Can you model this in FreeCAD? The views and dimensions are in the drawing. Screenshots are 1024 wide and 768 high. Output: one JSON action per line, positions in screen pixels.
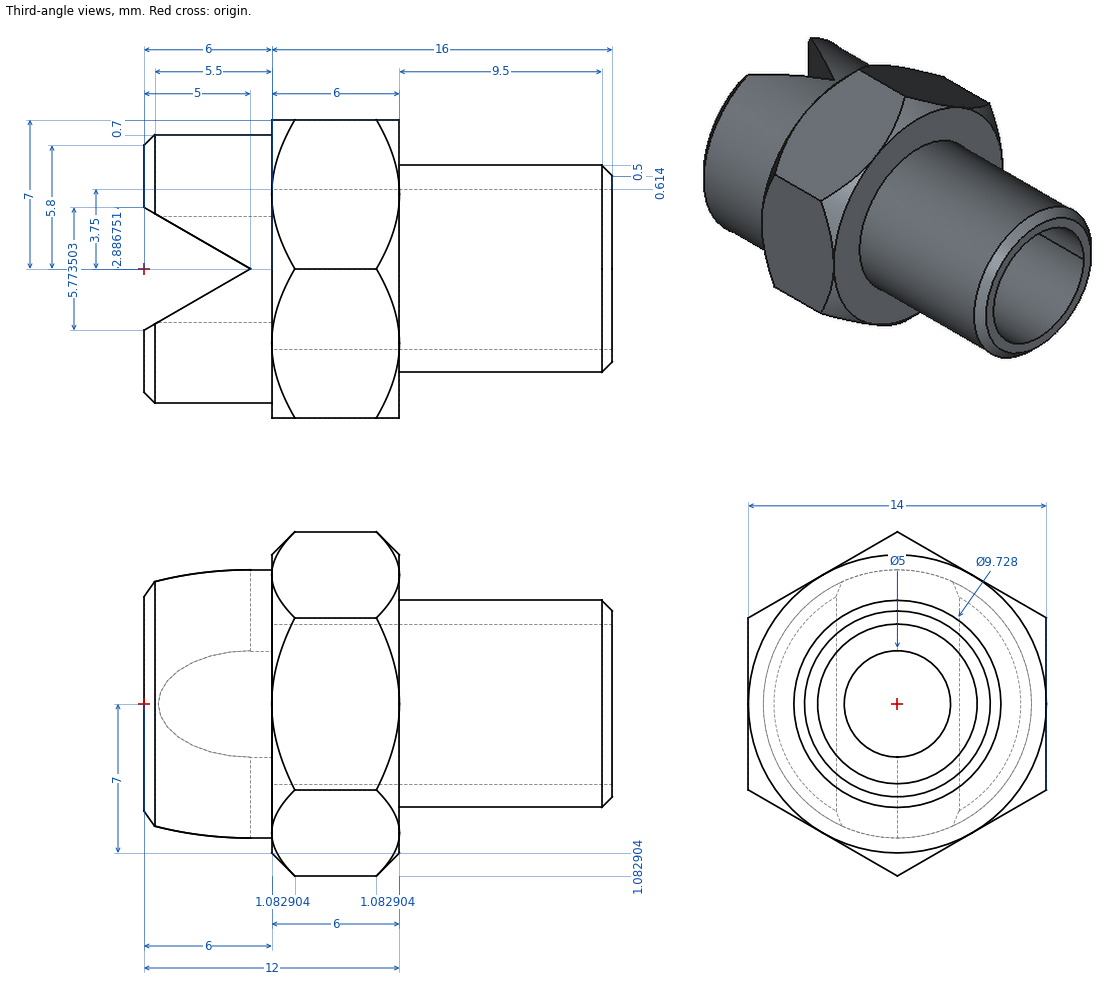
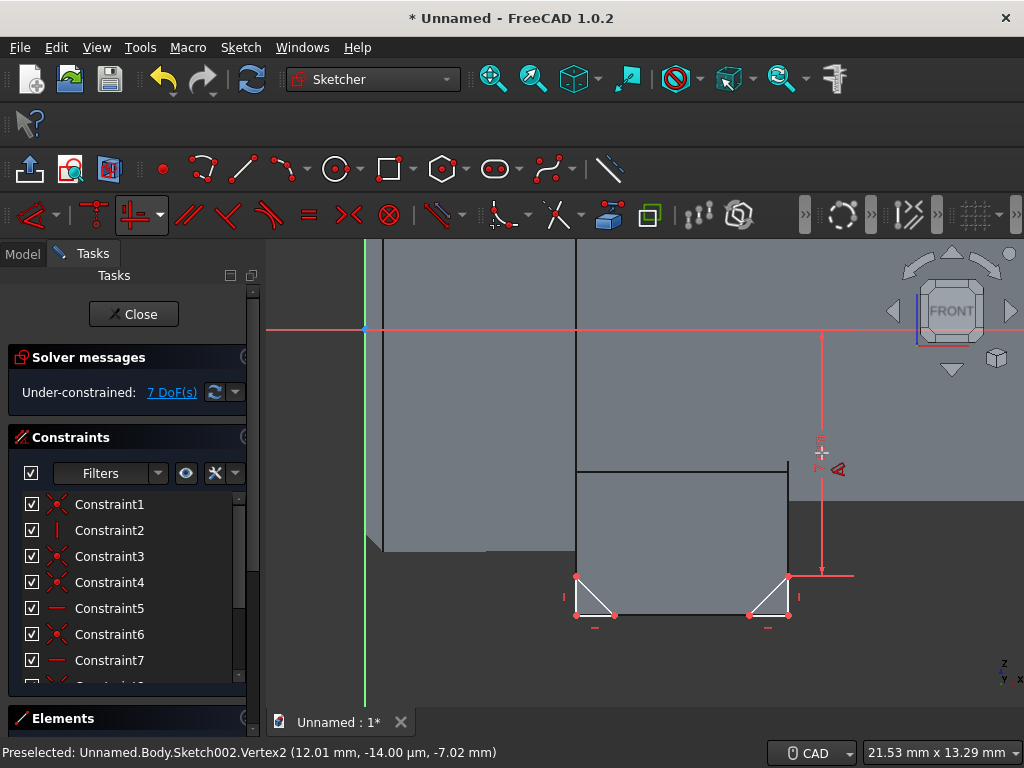
{"action": "left_click", "coordinate": [576, 577]}
{"action": "left_click", "coordinate": [471, 296]}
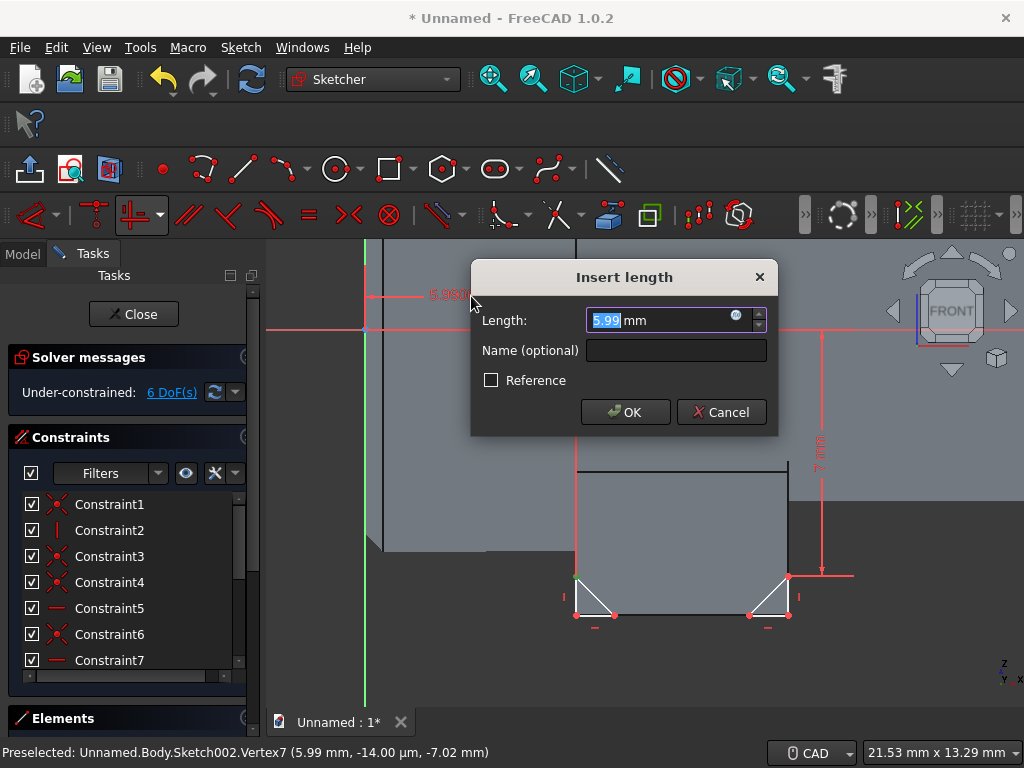
{"action": "type", "text": "6"}
{"action": "key", "text": "Return"}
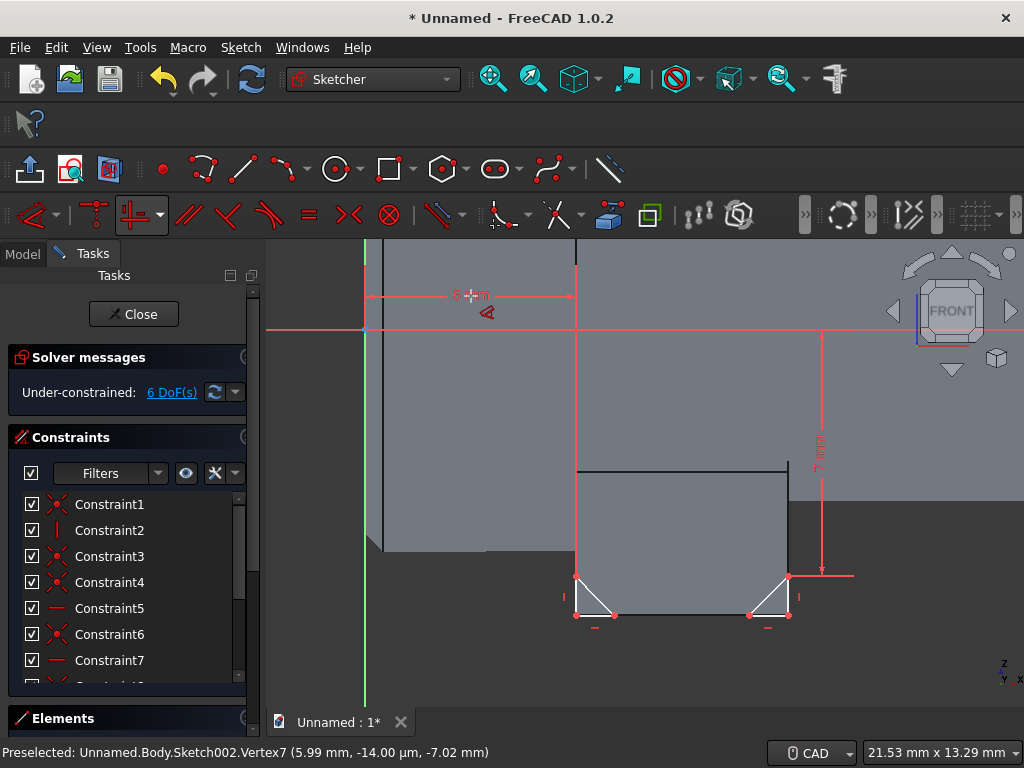
{"action": "left_click", "coordinate": [576, 577]}
{"action": "left_click", "coordinate": [331, 453]}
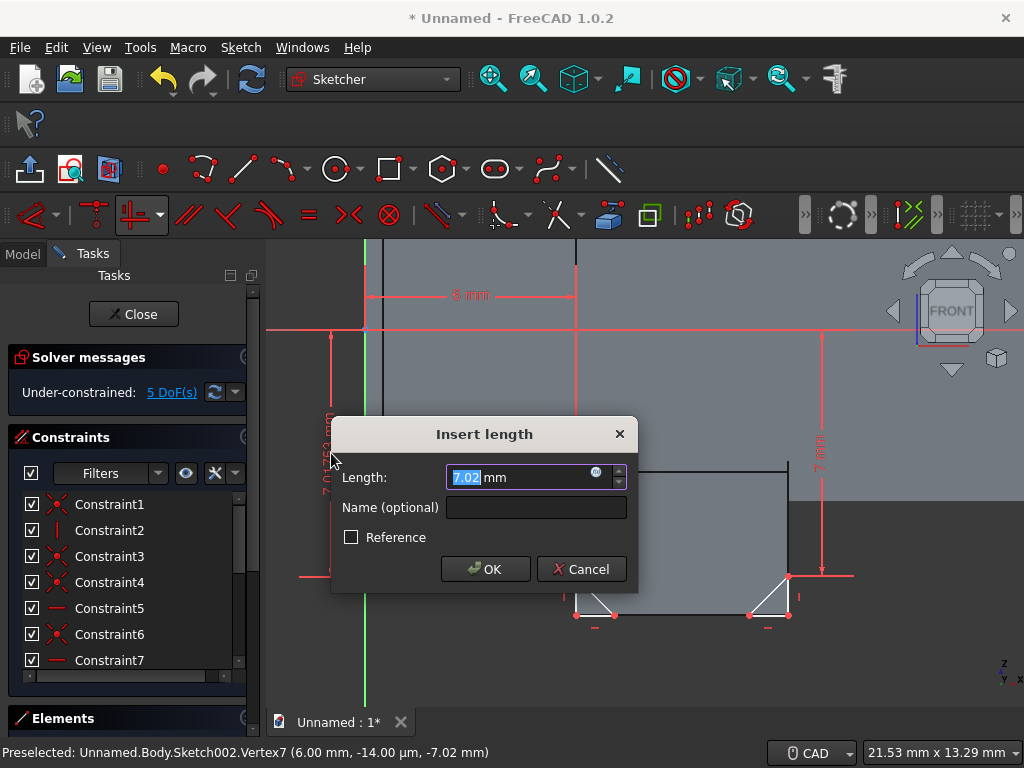
{"action": "type", "text": "7"}
{"action": "key", "text": "Return"}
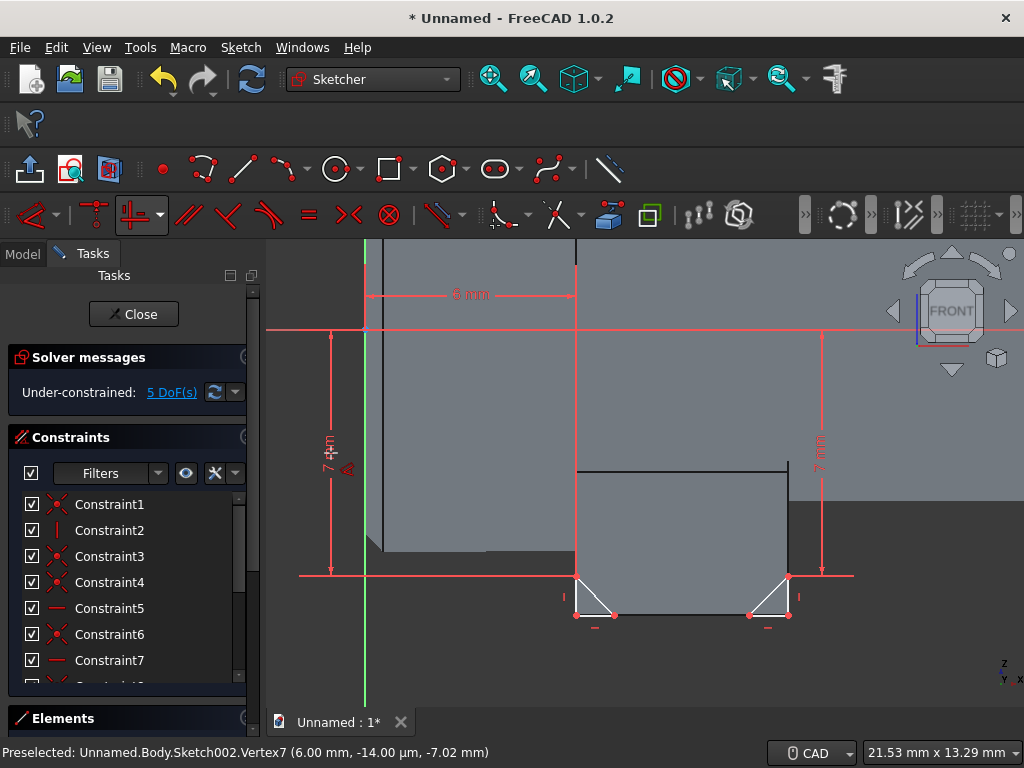
{"action": "left_click", "coordinate": [788, 576]}
{"action": "left_click", "coordinate": [577, 296]}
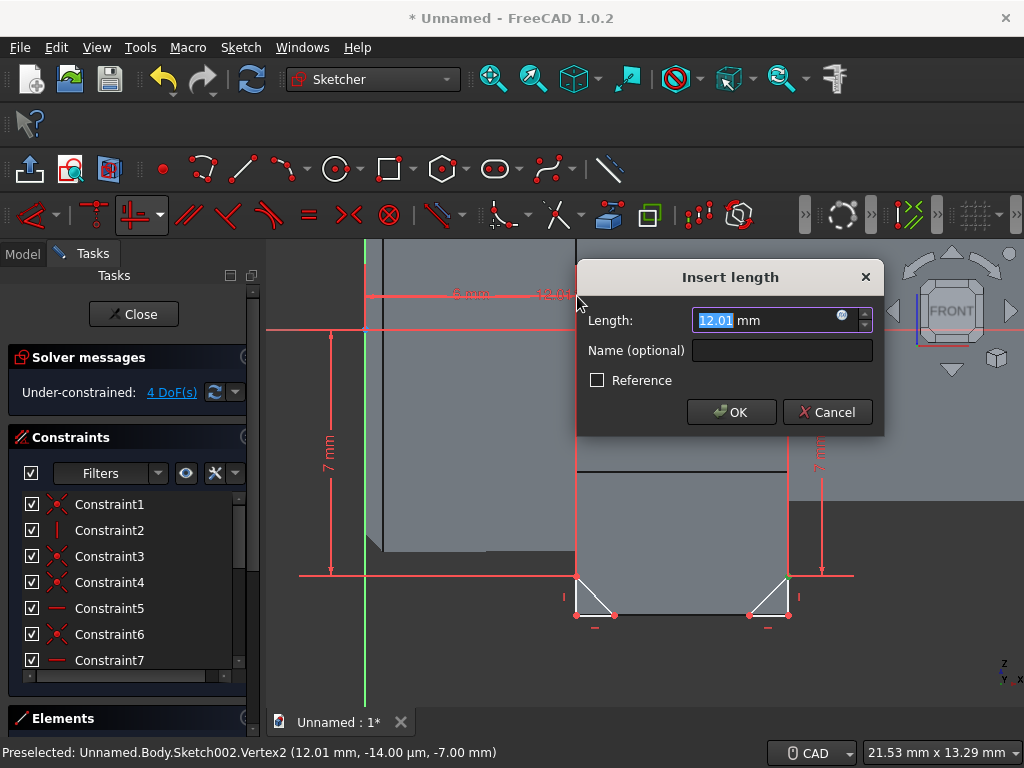
{"action": "type", "text": "12"}
{"action": "key", "text": "Return"}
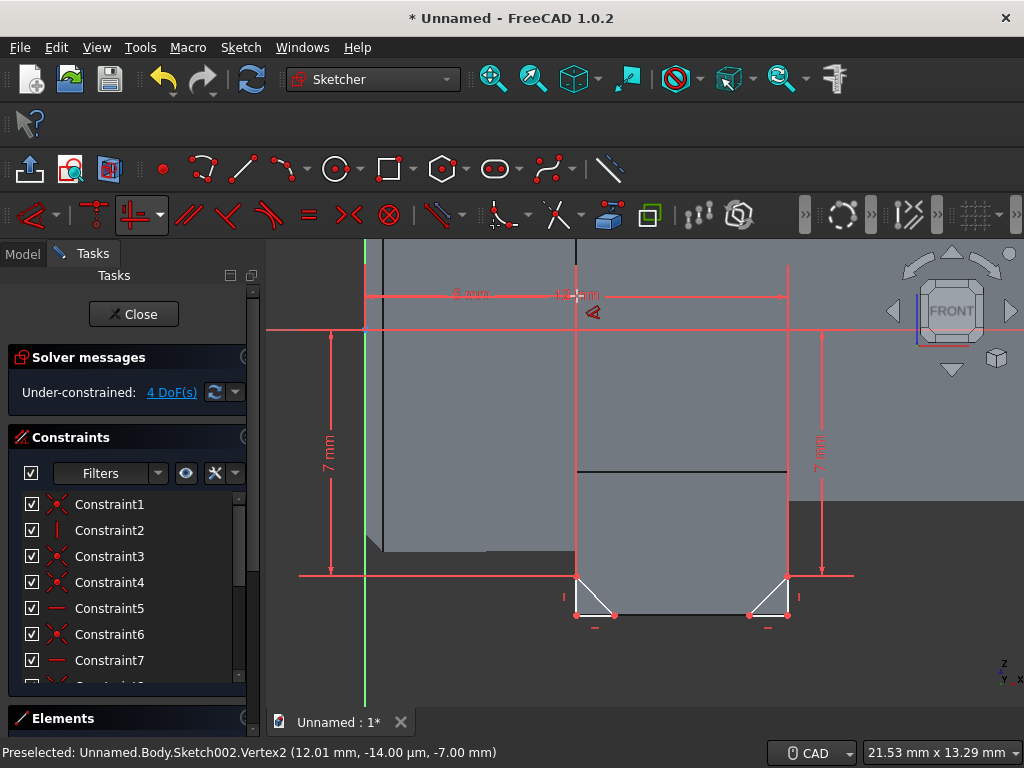
{"action": "left_click", "coordinate": [788, 604]}
{"action": "left_click", "coordinate": [822, 596]}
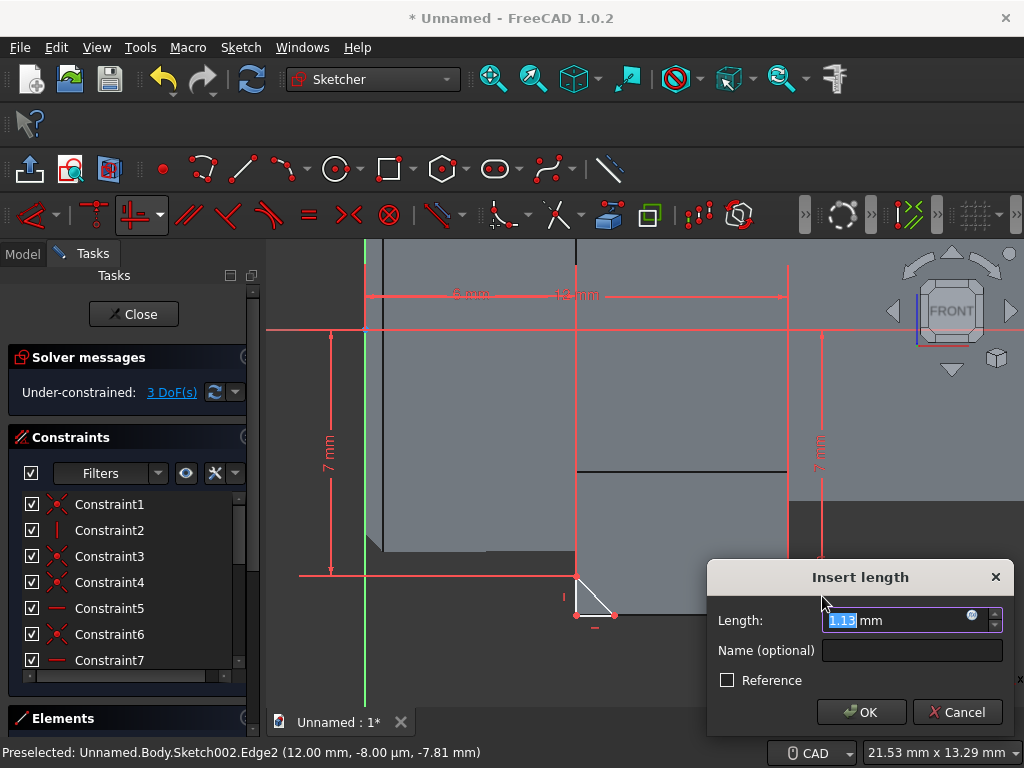
{"action": "type", "text": "1.082904"}
{"action": "key", "text": "Return"}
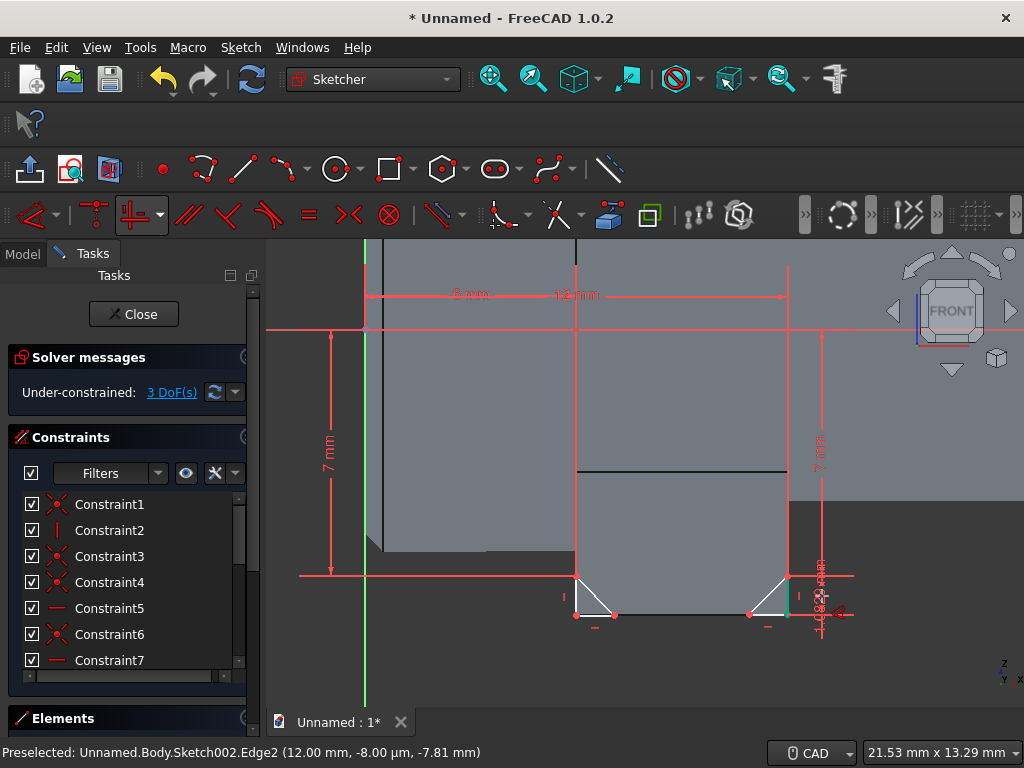
{"action": "left_click", "coordinate": [776, 615]}
{"action": "left_click", "coordinate": [768, 649]}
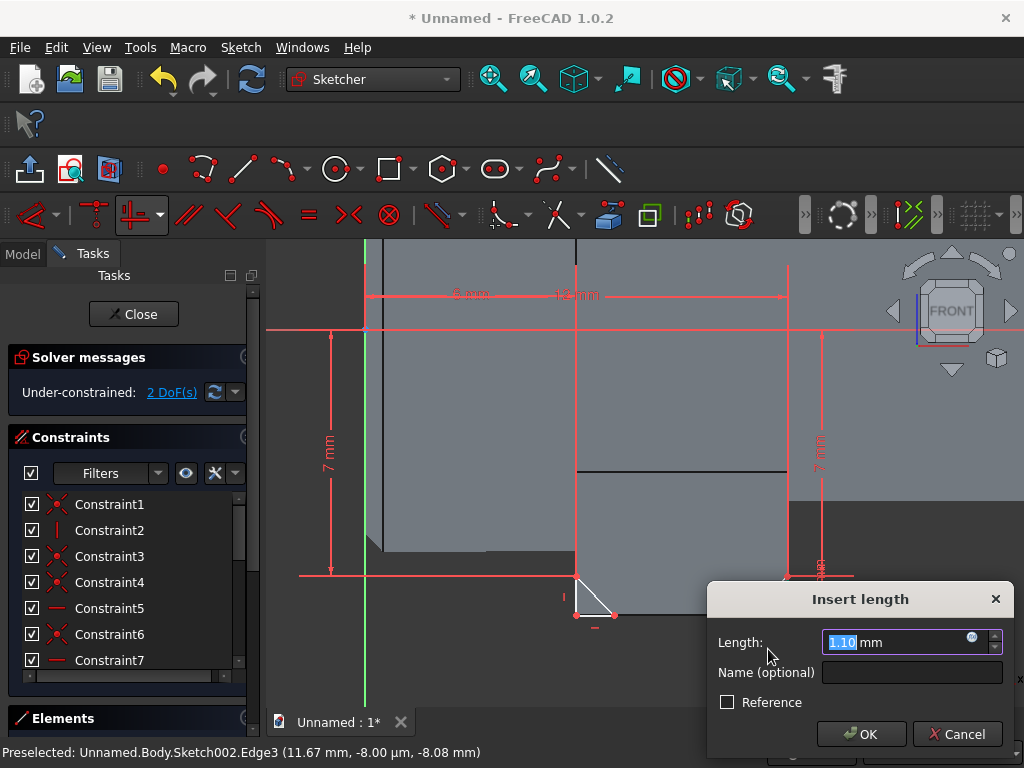
{"action": "type", "text": "1.082904"}
{"action": "key", "text": "Return"}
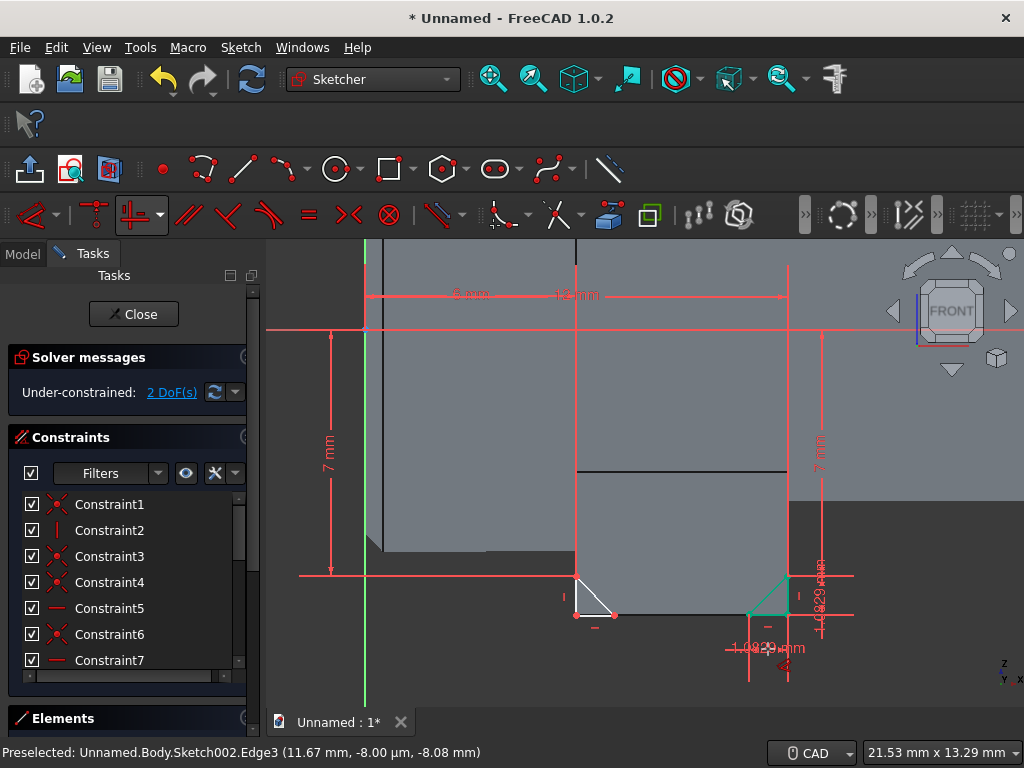
{"action": "scroll", "coordinate": [588, 616], "scroll_direction": "up", "scroll_amount": 2}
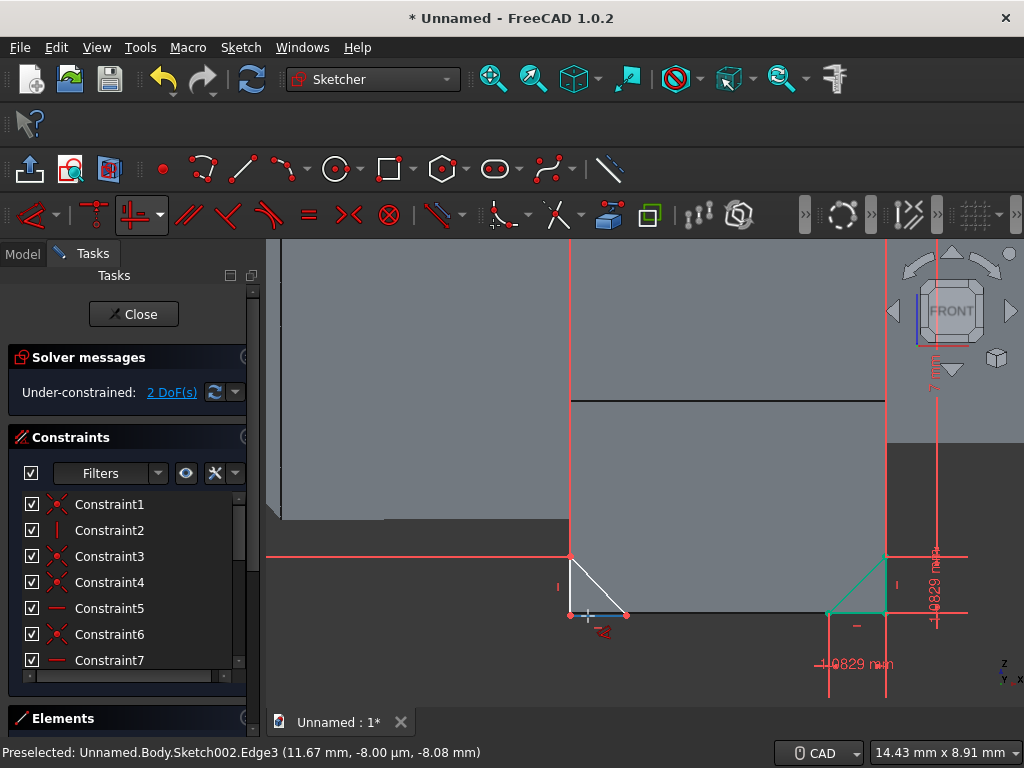
{"action": "left_click", "coordinate": [587, 616]}
{"action": "left_click", "coordinate": [598, 650]}